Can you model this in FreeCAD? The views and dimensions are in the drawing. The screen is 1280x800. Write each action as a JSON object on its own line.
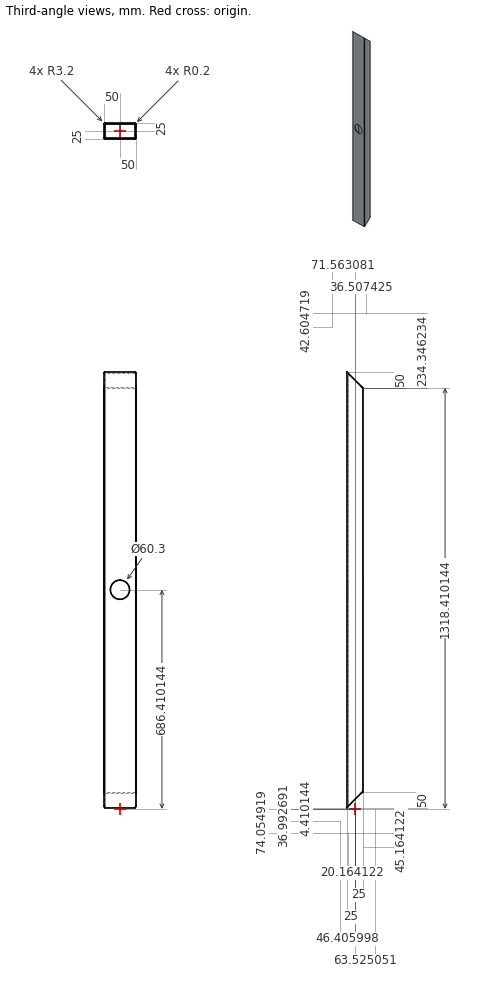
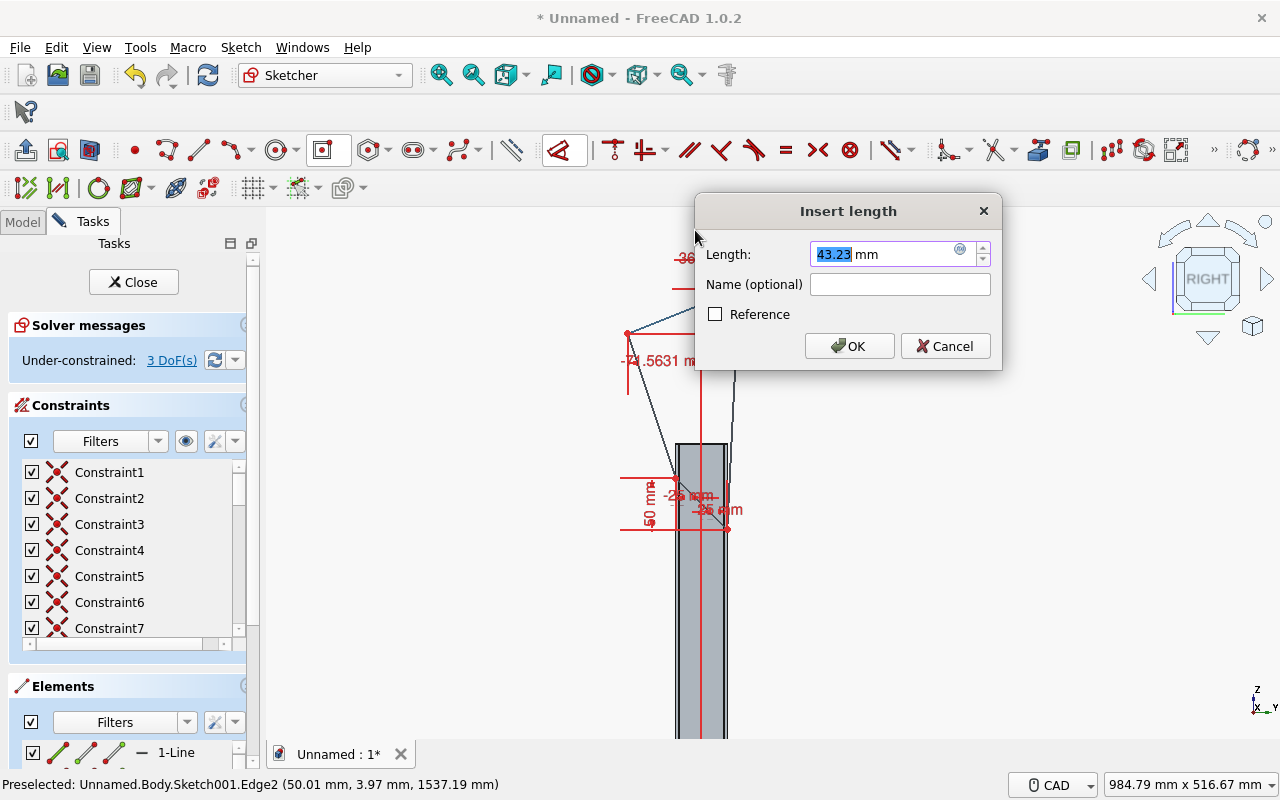
{"action": "type", "text": "42.604719"}
{"action": "key", "text": "Return"}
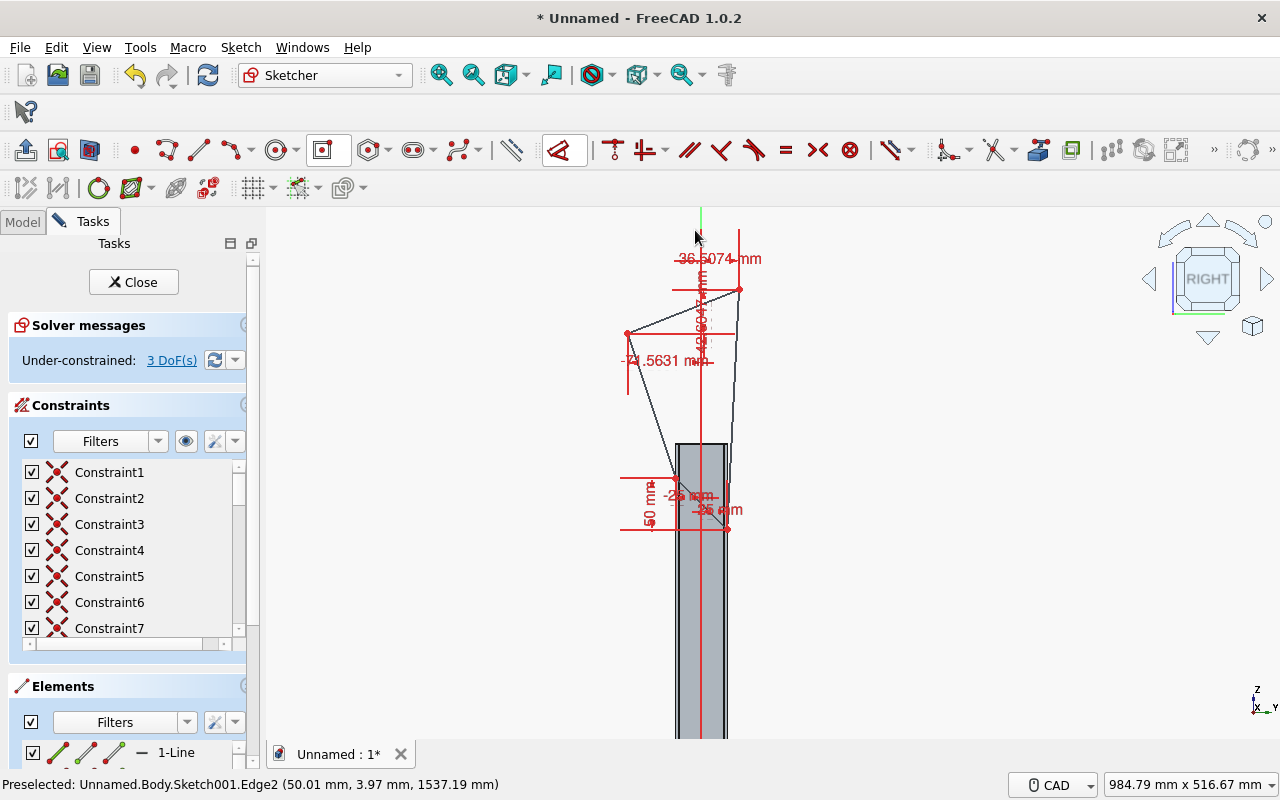
{"action": "scroll", "coordinate": [706, 302], "scroll_direction": "down", "scroll_amount": 8}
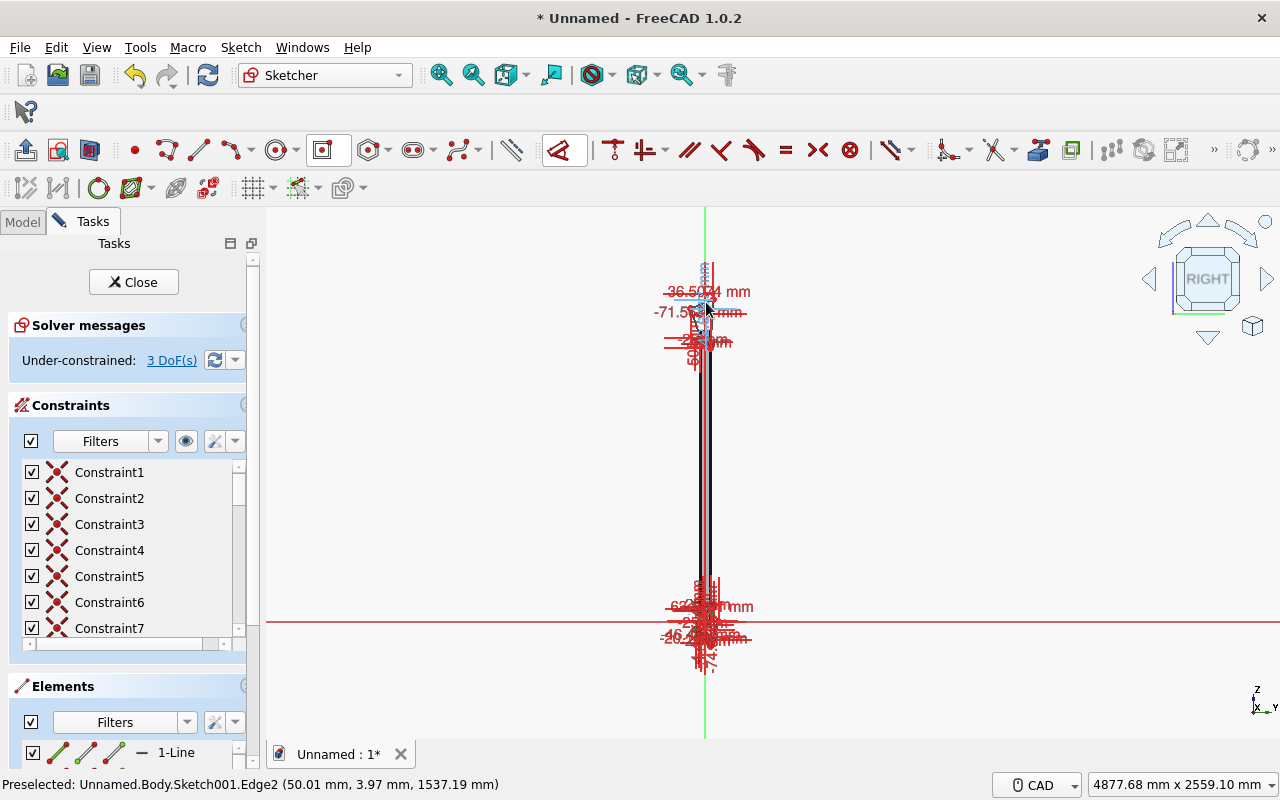
{"action": "scroll", "coordinate": [708, 644], "scroll_direction": "up", "scroll_amount": 9}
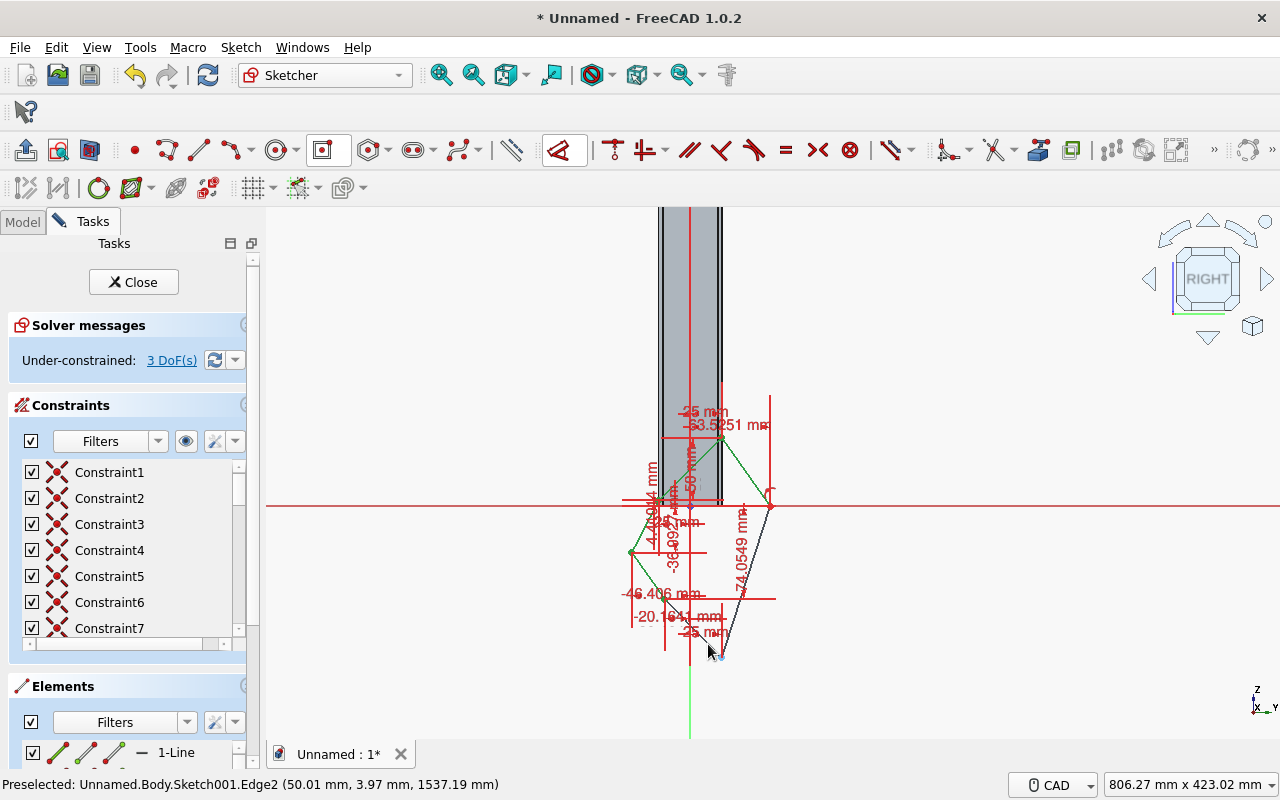
{"action": "left_click", "coordinate": [710, 646]}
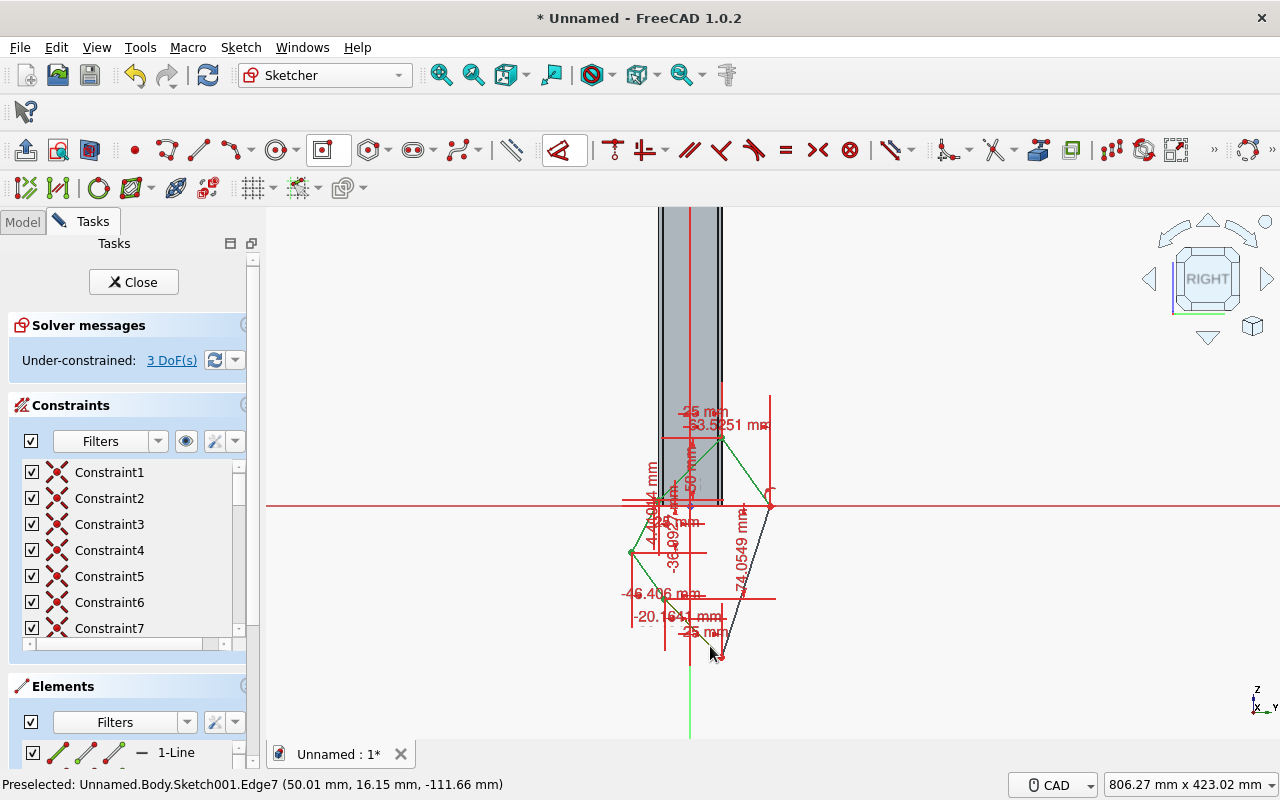
{"action": "left_click", "coordinate": [582, 150]}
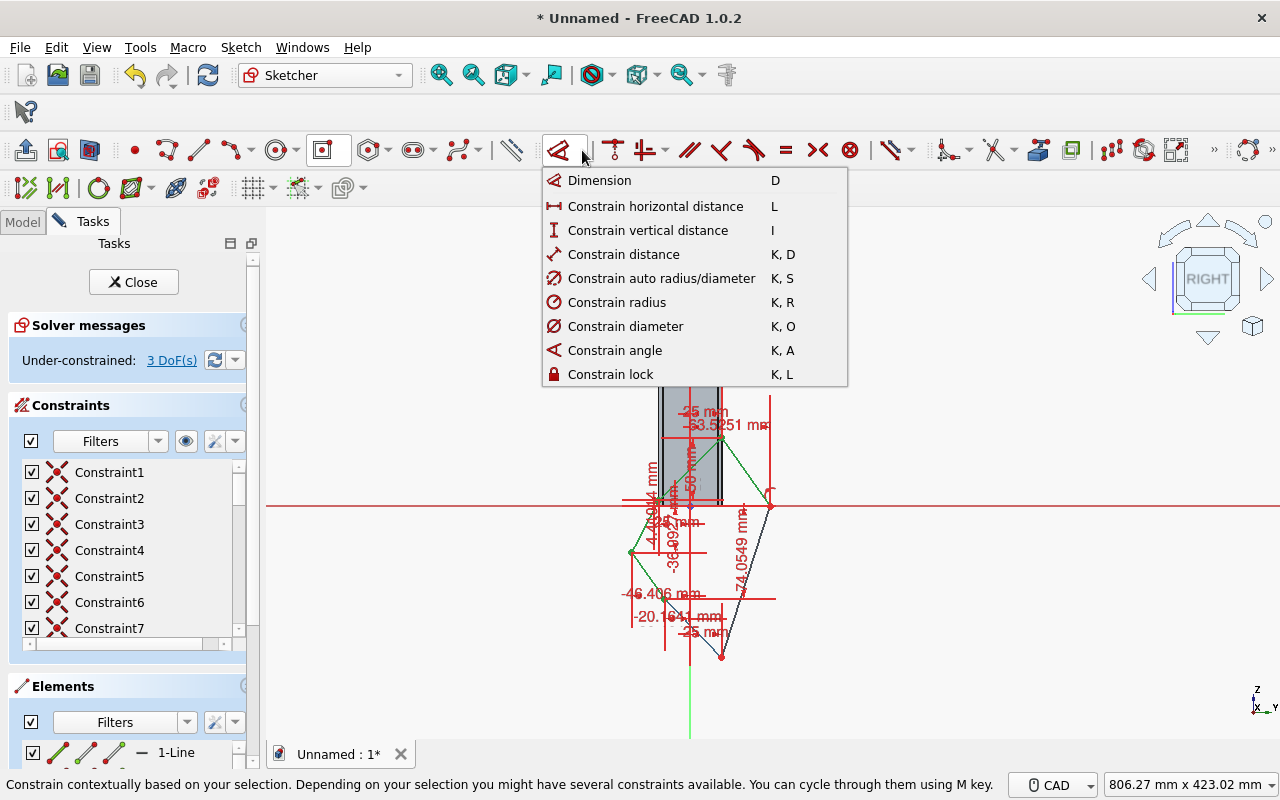
{"action": "left_click", "coordinate": [695, 230]}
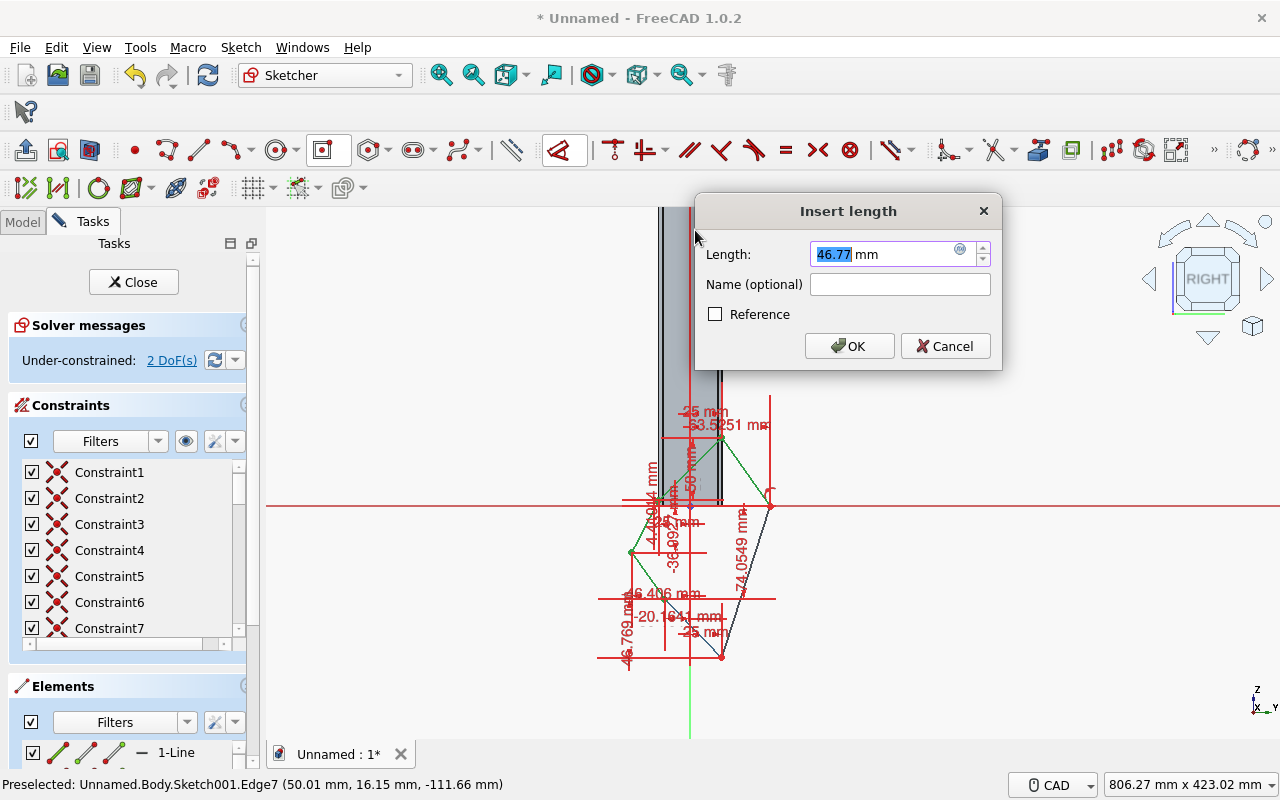
{"action": "type", "text": "45.164122"}
{"action": "key", "text": "Return"}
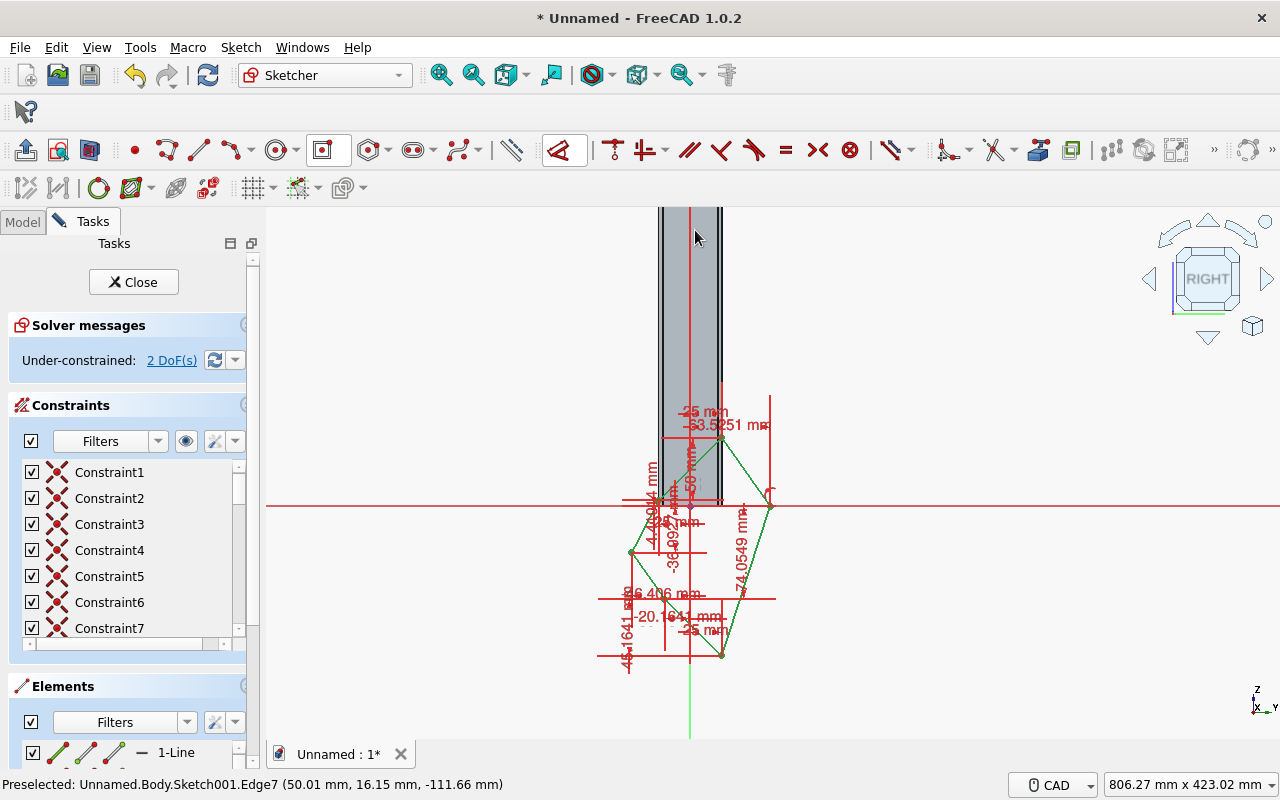
{"action": "scroll", "coordinate": [708, 645], "scroll_direction": "down", "scroll_amount": 9}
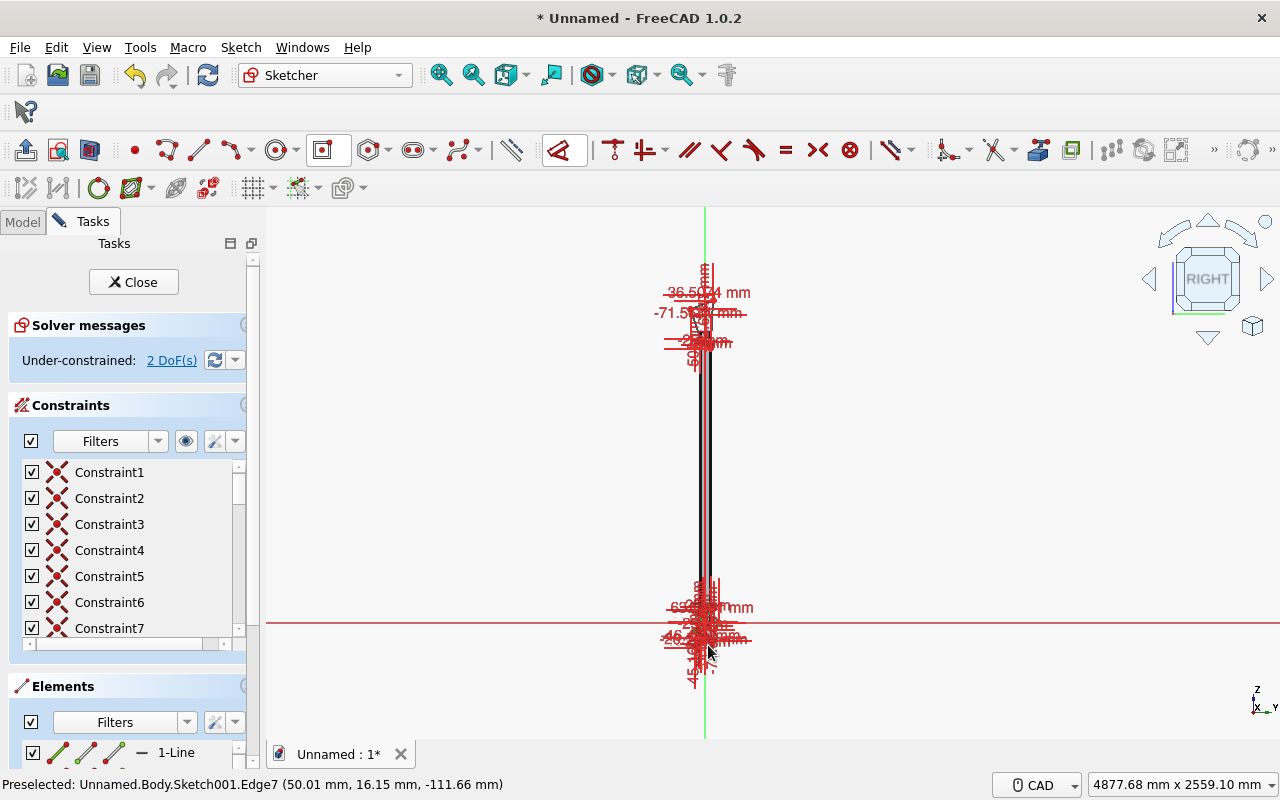
{"action": "scroll", "coordinate": [711, 334], "scroll_direction": "up", "scroll_amount": 5}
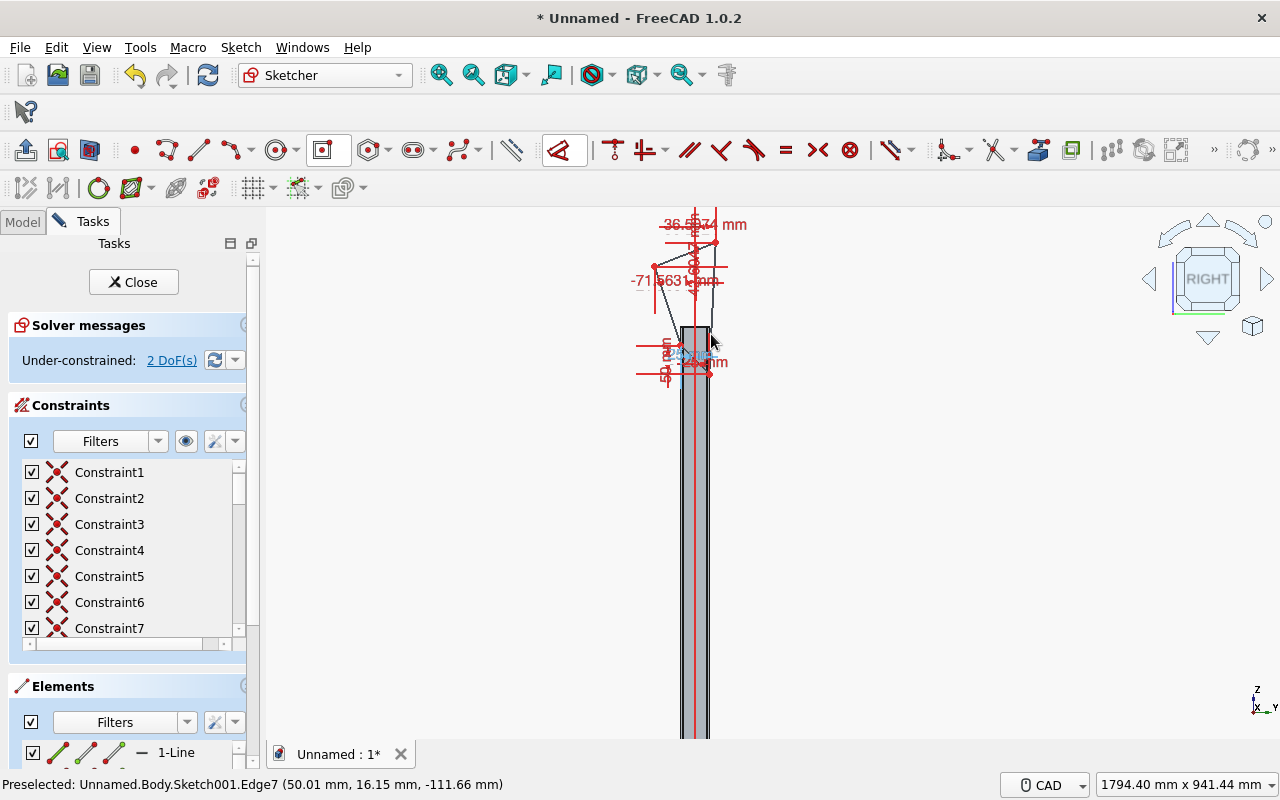
{"action": "left_click", "coordinate": [711, 335]}